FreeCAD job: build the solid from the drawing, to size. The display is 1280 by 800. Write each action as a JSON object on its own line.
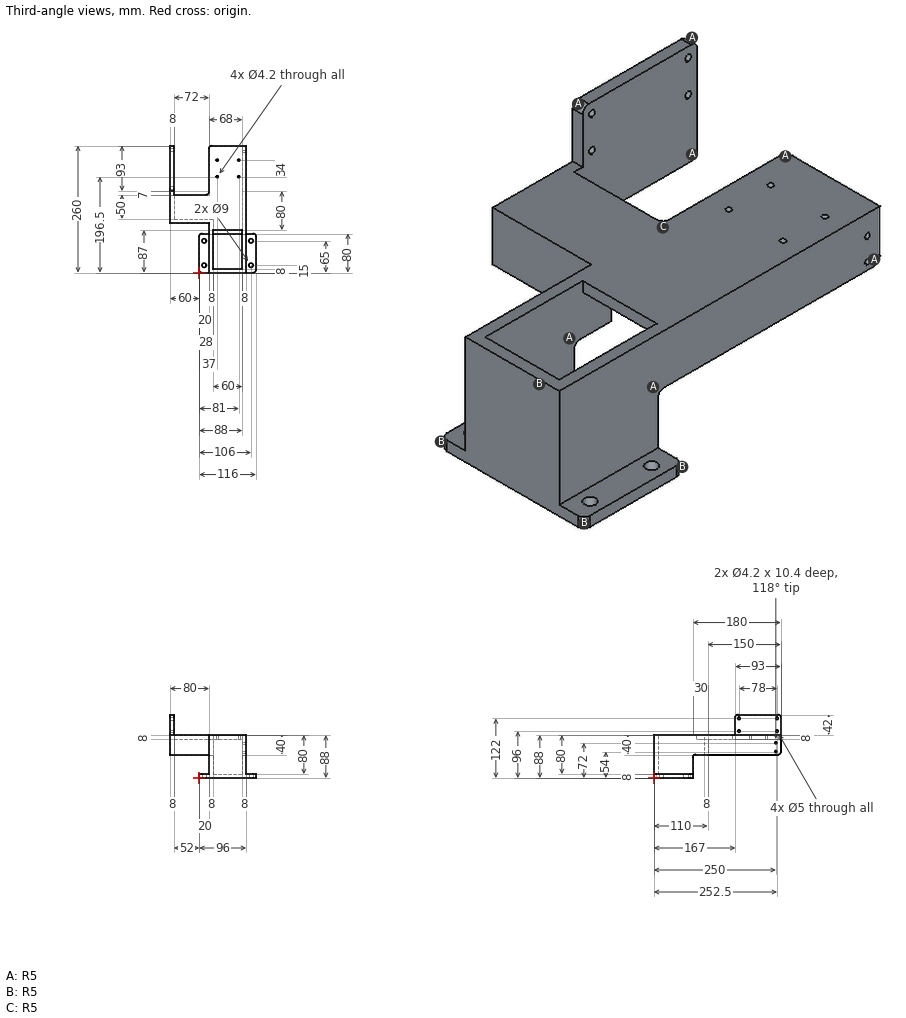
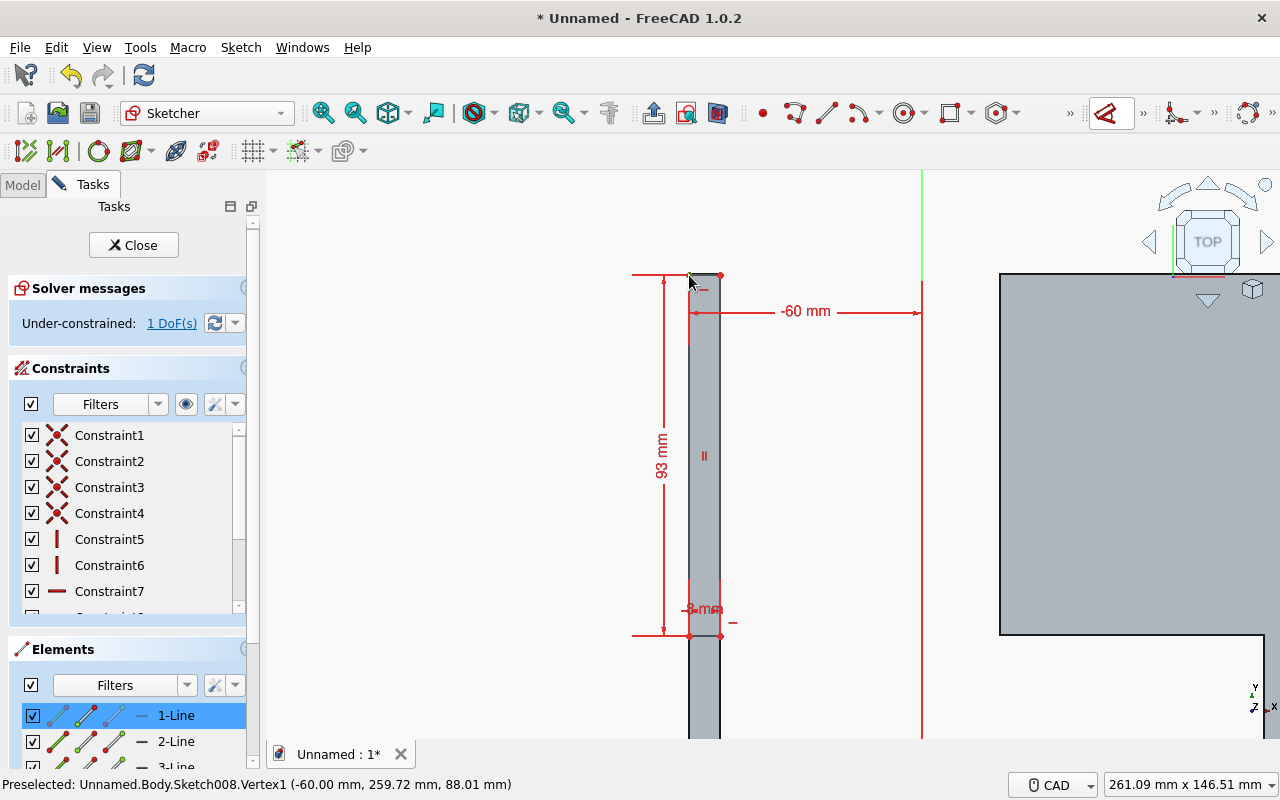
{"action": "left_click", "coordinate": [1128, 114]}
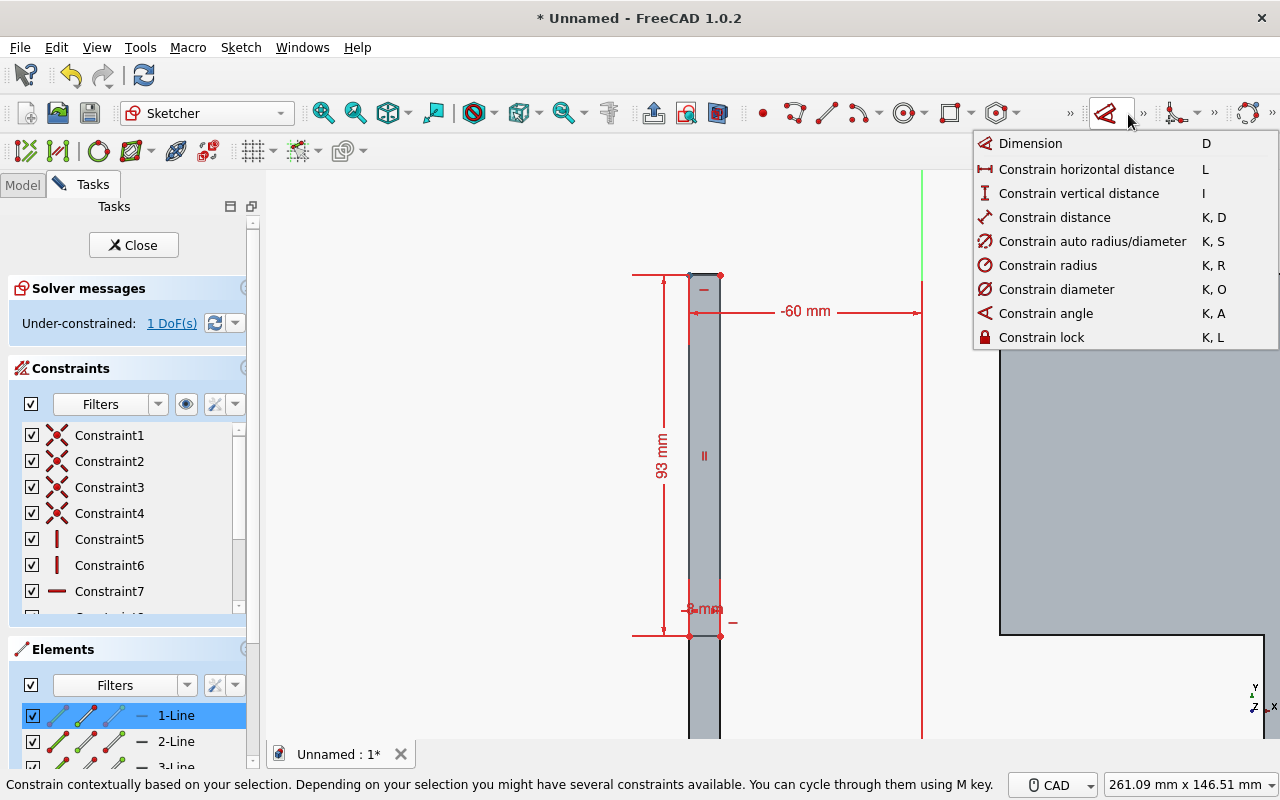
{"action": "left_click", "coordinate": [1126, 193]}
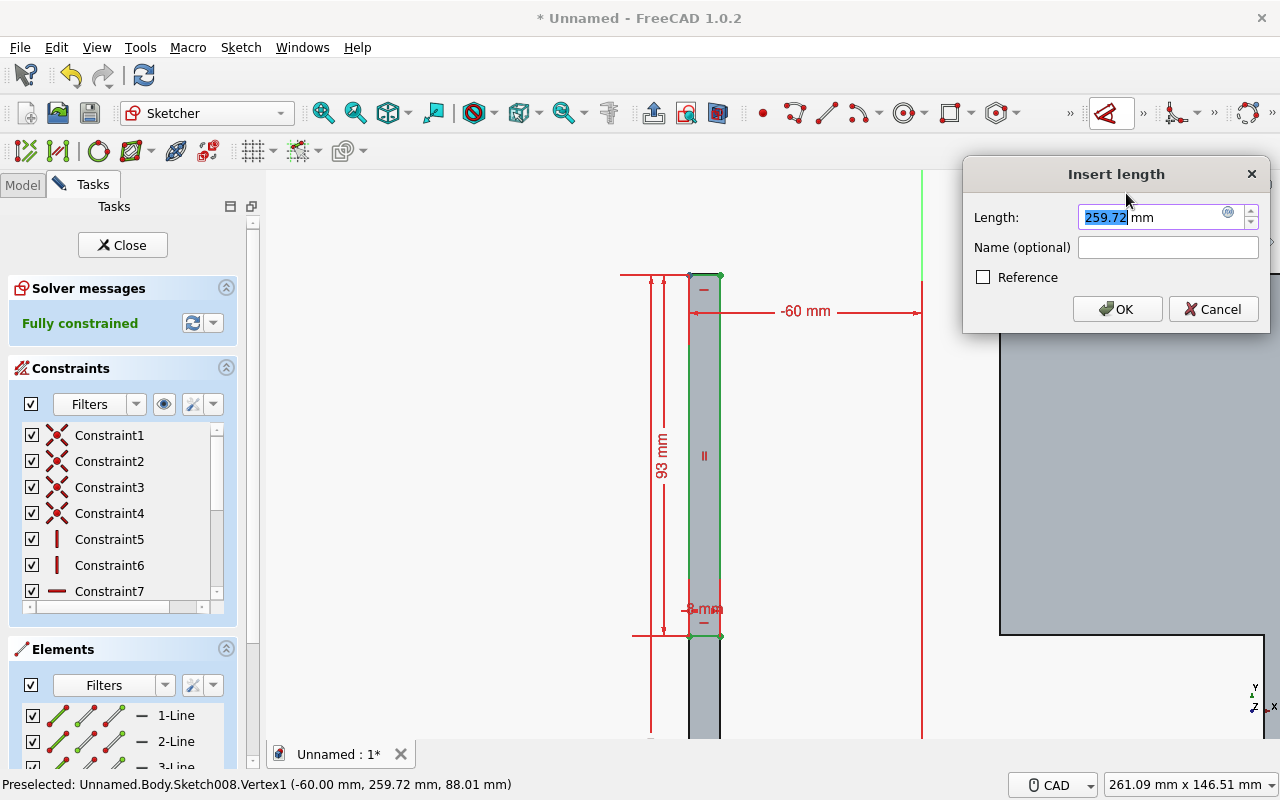
{"action": "type", "text": "260"}
{"action": "key", "text": "Return"}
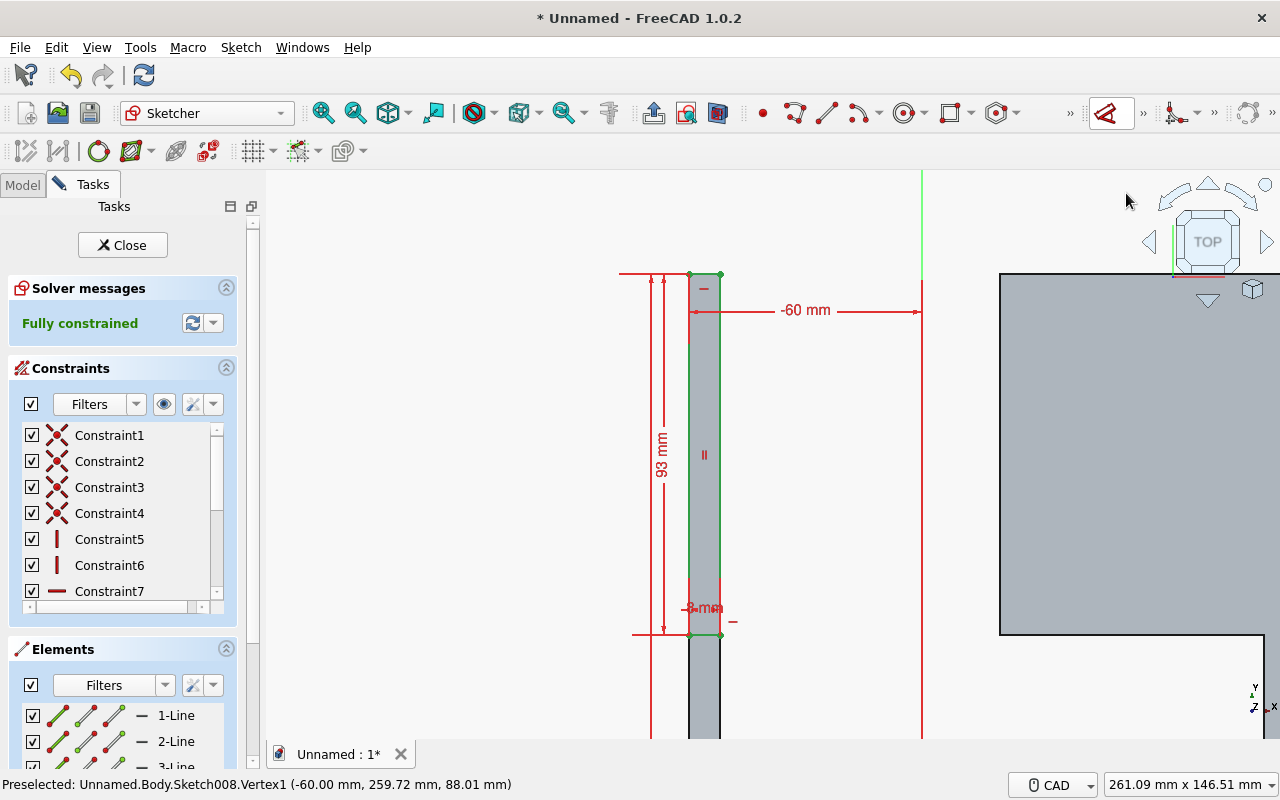
{"action": "left_click", "coordinate": [123, 245]}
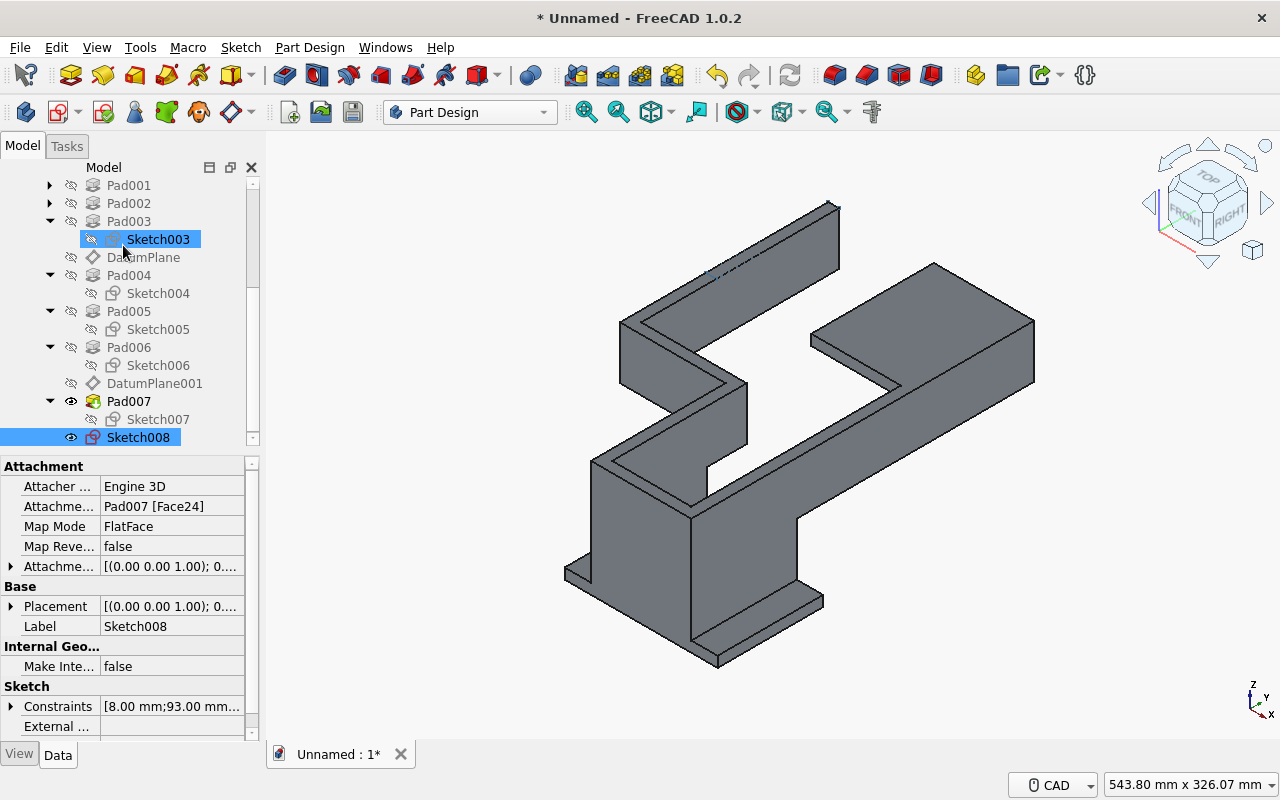
{"action": "left_click", "coordinate": [72, 76]}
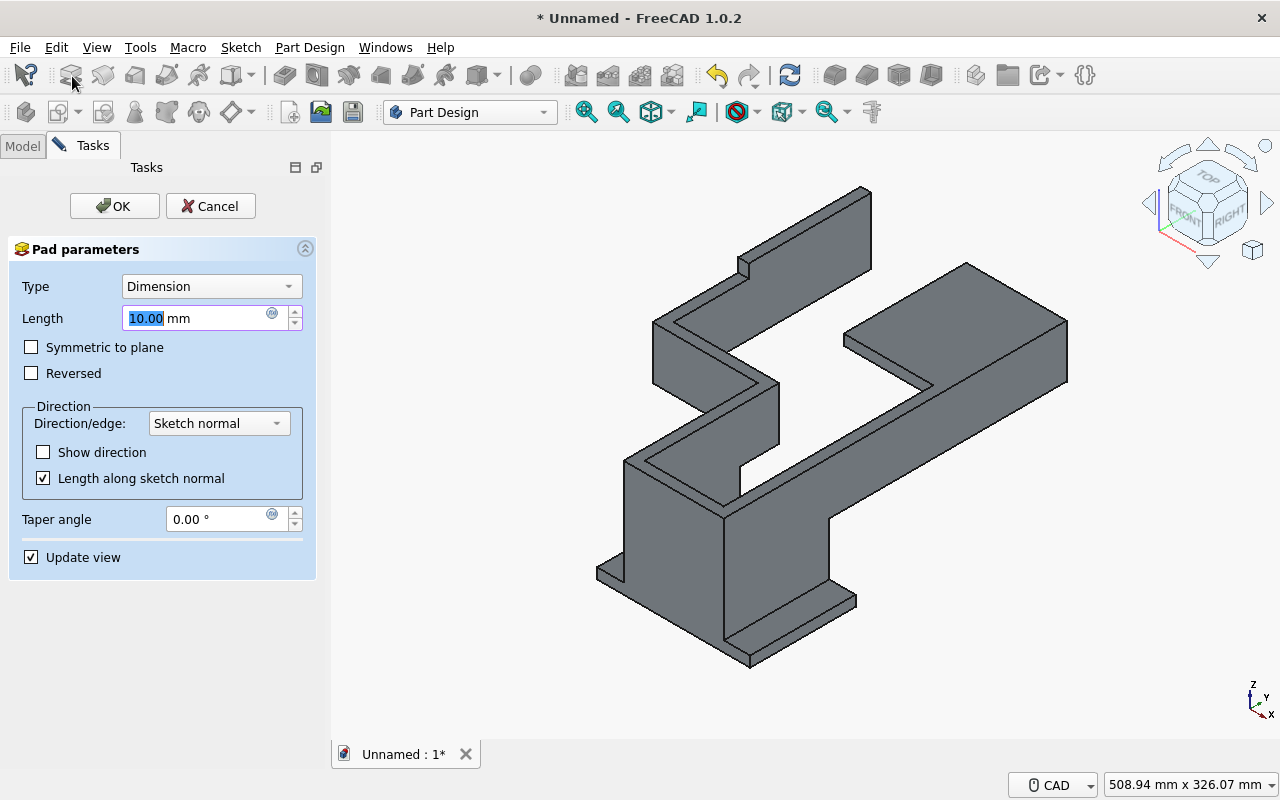
{"action": "type", "text": "42"}
{"action": "key", "text": "Tab"}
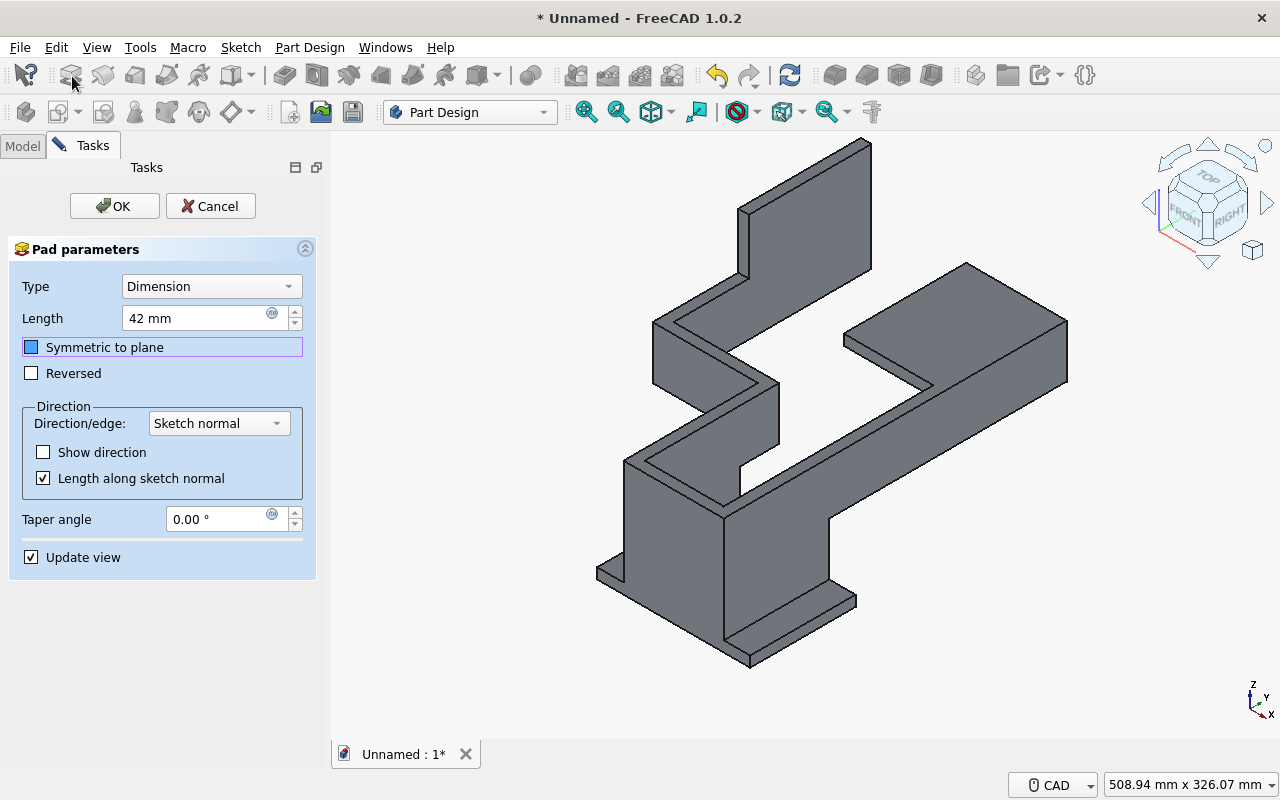
{"action": "left_click", "coordinate": [115, 206]}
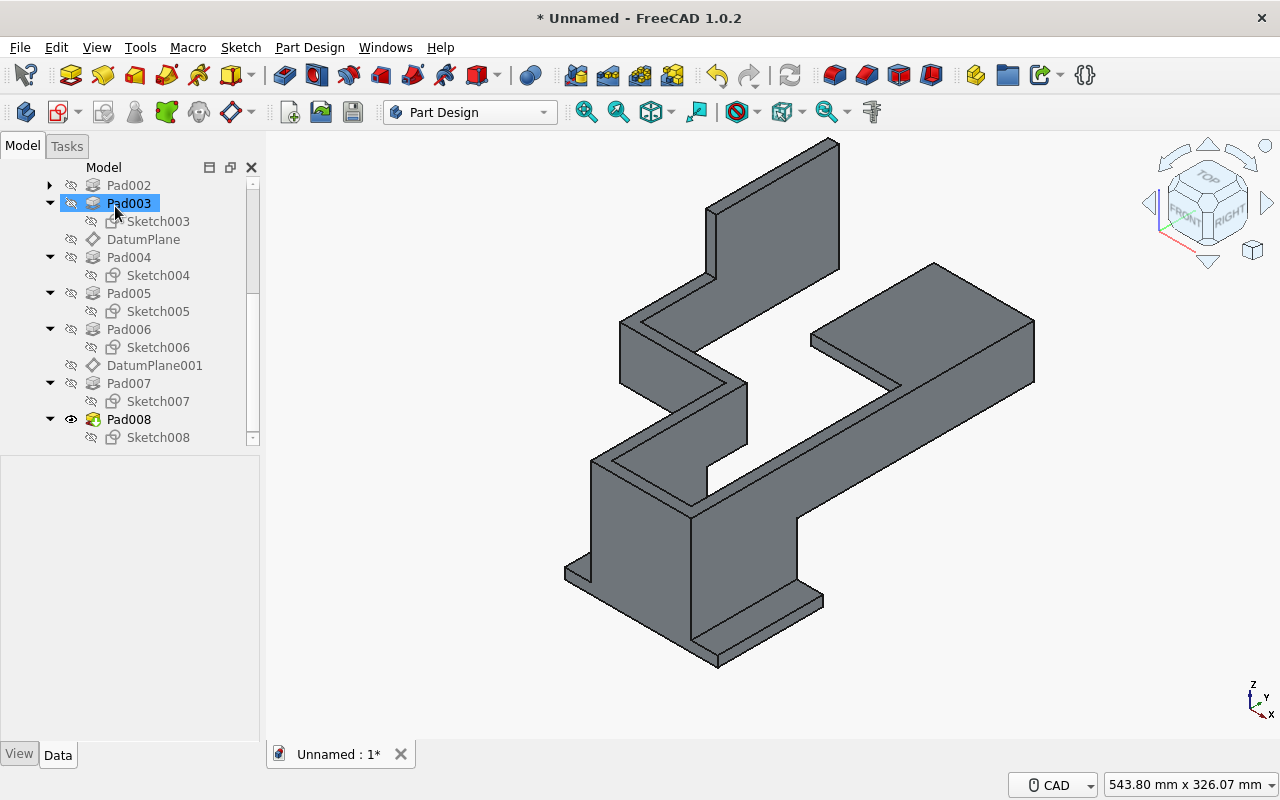
{"action": "left_click", "coordinate": [710, 210]}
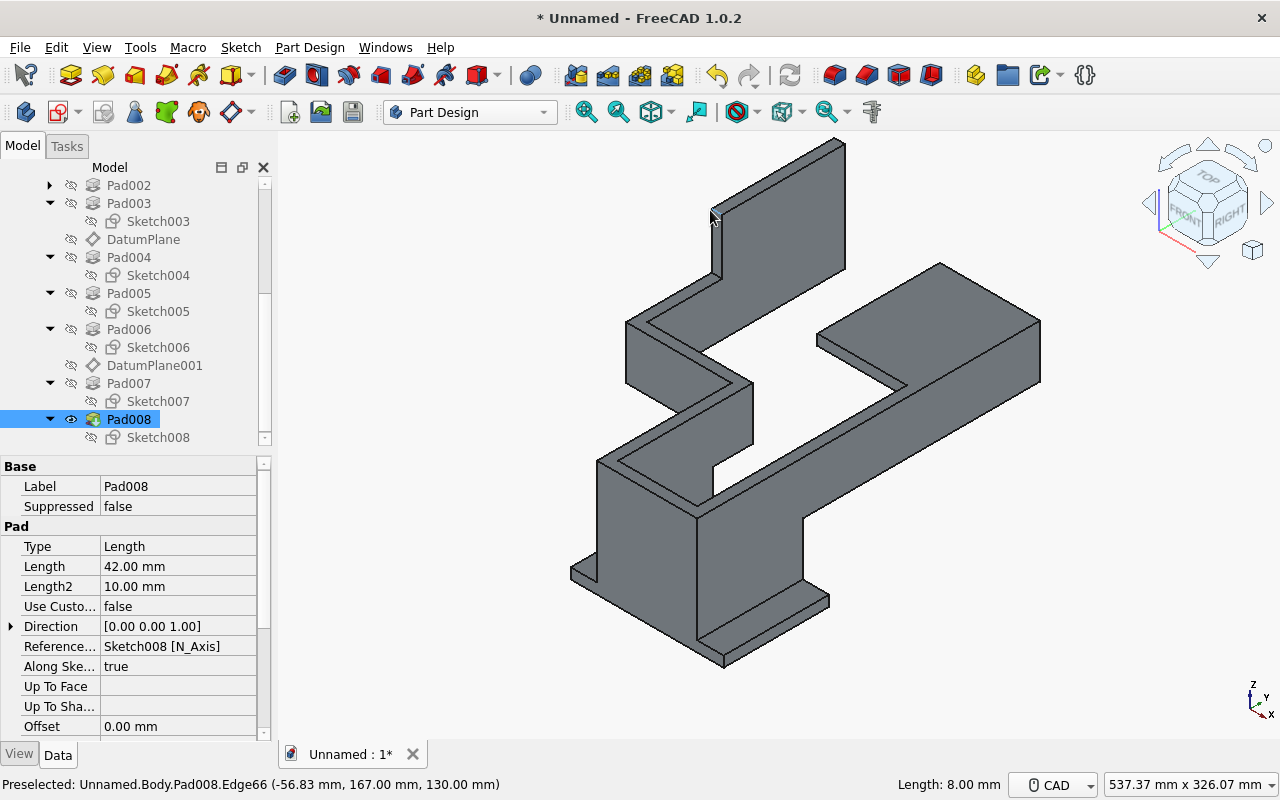
{"action": "scroll", "coordinate": [840, 265], "scroll_direction": "up", "scroll_amount": 5}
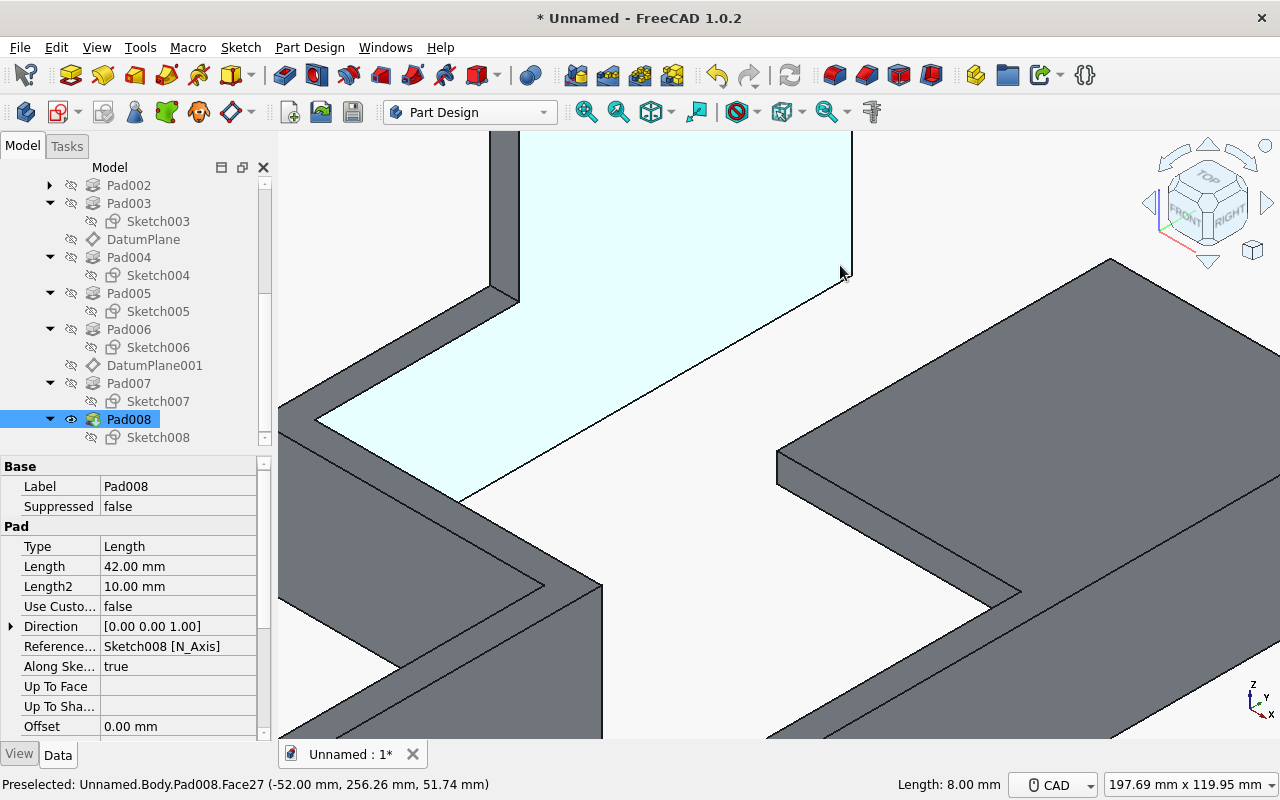
{"action": "left_click", "coordinate": [588, 112]}